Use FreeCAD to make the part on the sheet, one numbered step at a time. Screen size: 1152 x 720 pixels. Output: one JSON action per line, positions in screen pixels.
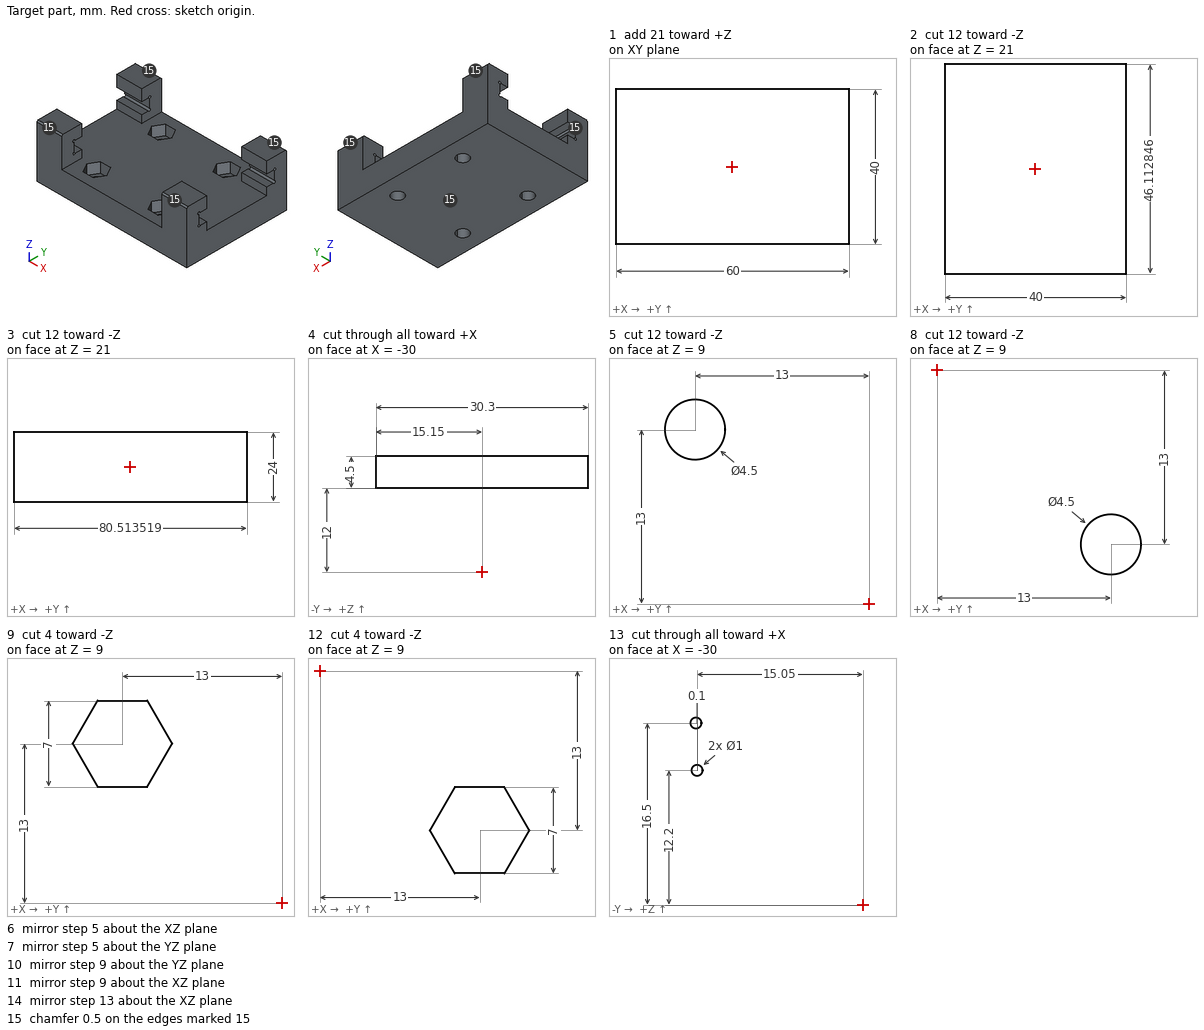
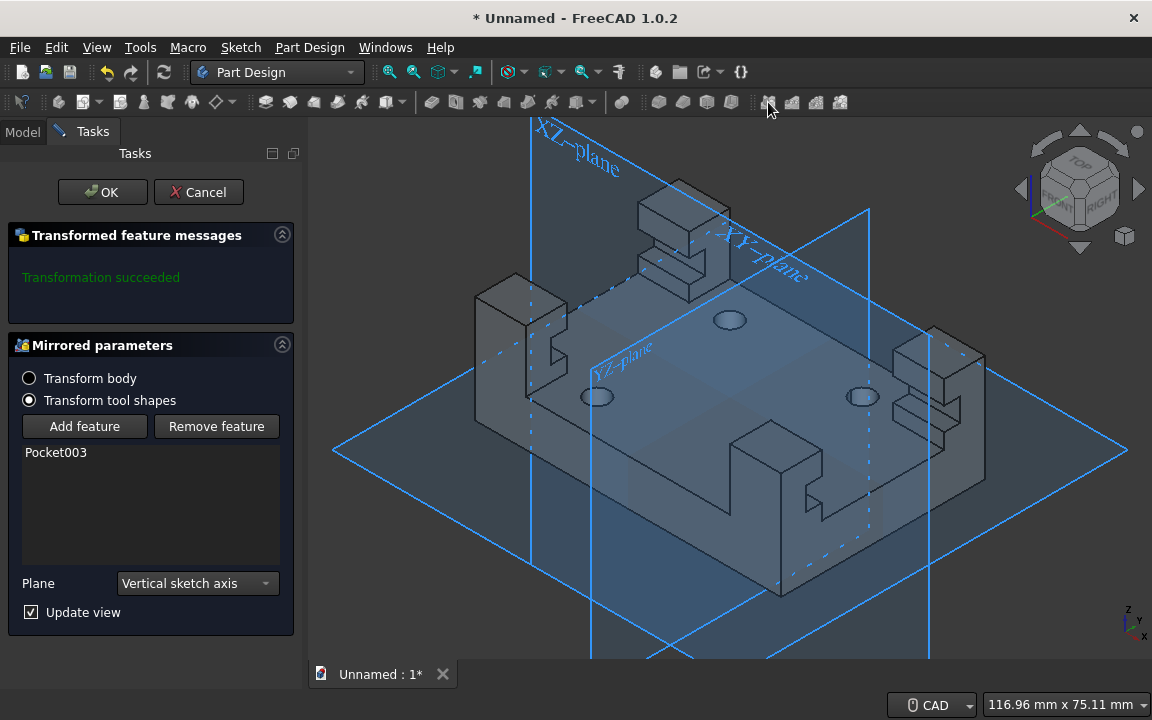
{"action": "left_click", "coordinate": [198, 584]}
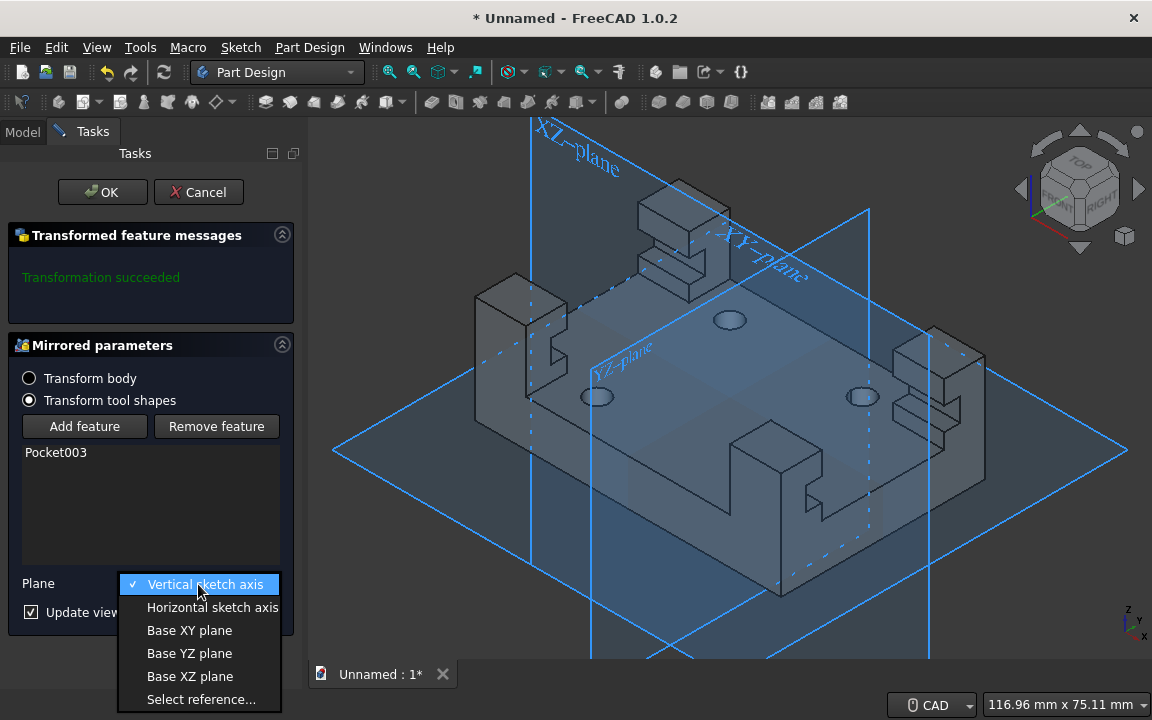
{"action": "left_click", "coordinate": [198, 654]}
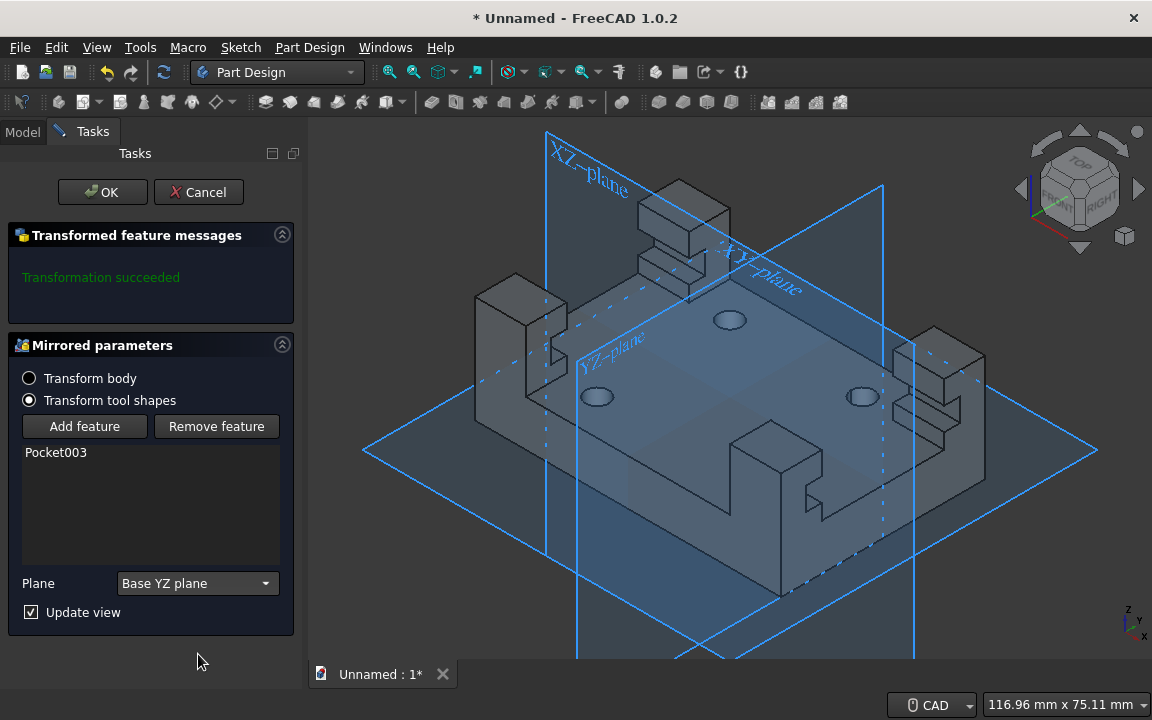
{"action": "left_click", "coordinate": [103, 192]}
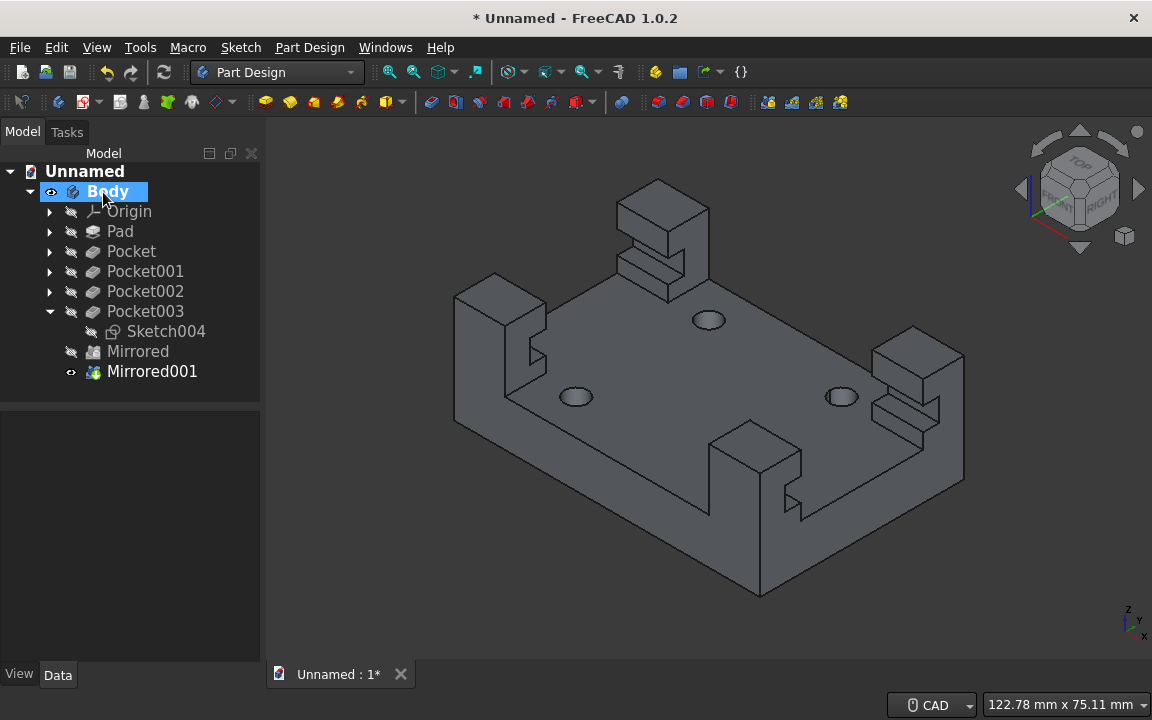
{"action": "left_click", "coordinate": [709, 396]}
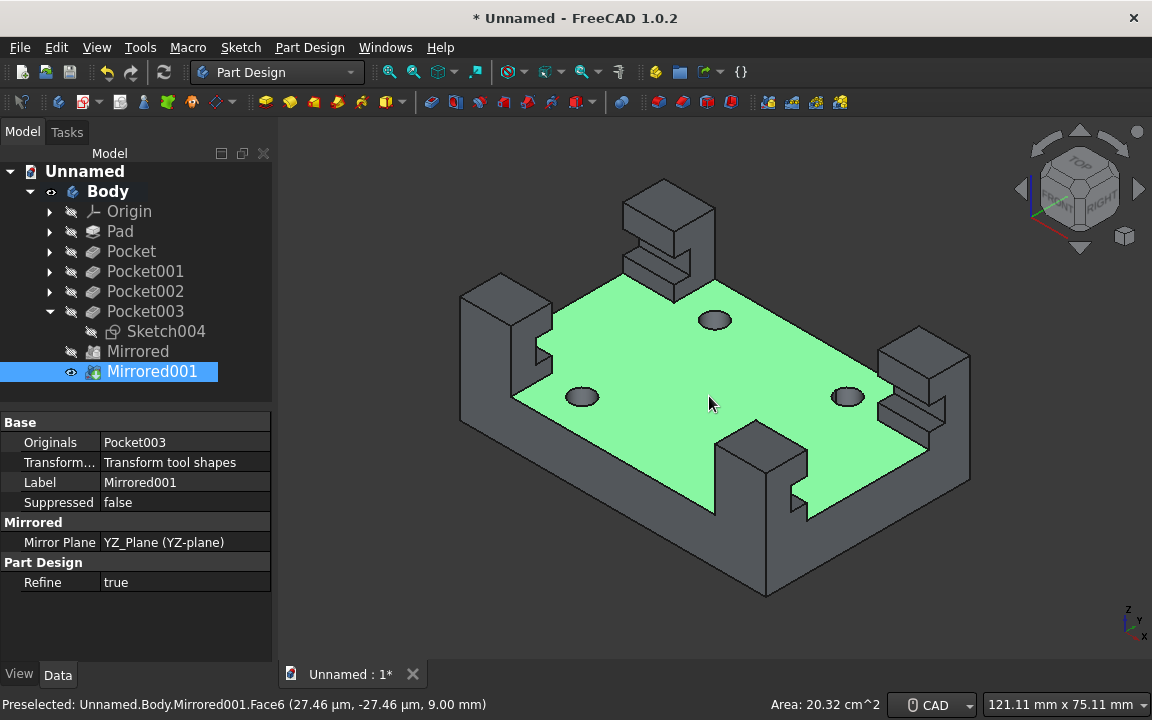
{"action": "left_click", "coordinate": [84, 102]}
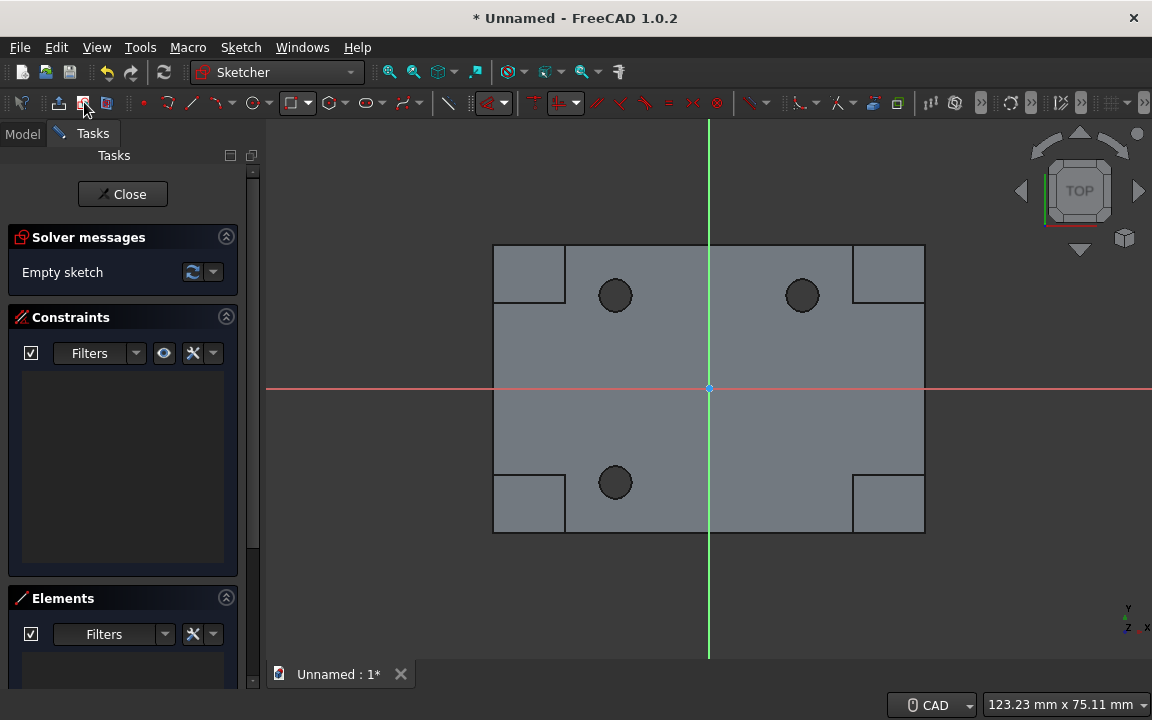
{"action": "left_click", "coordinate": [108, 104]}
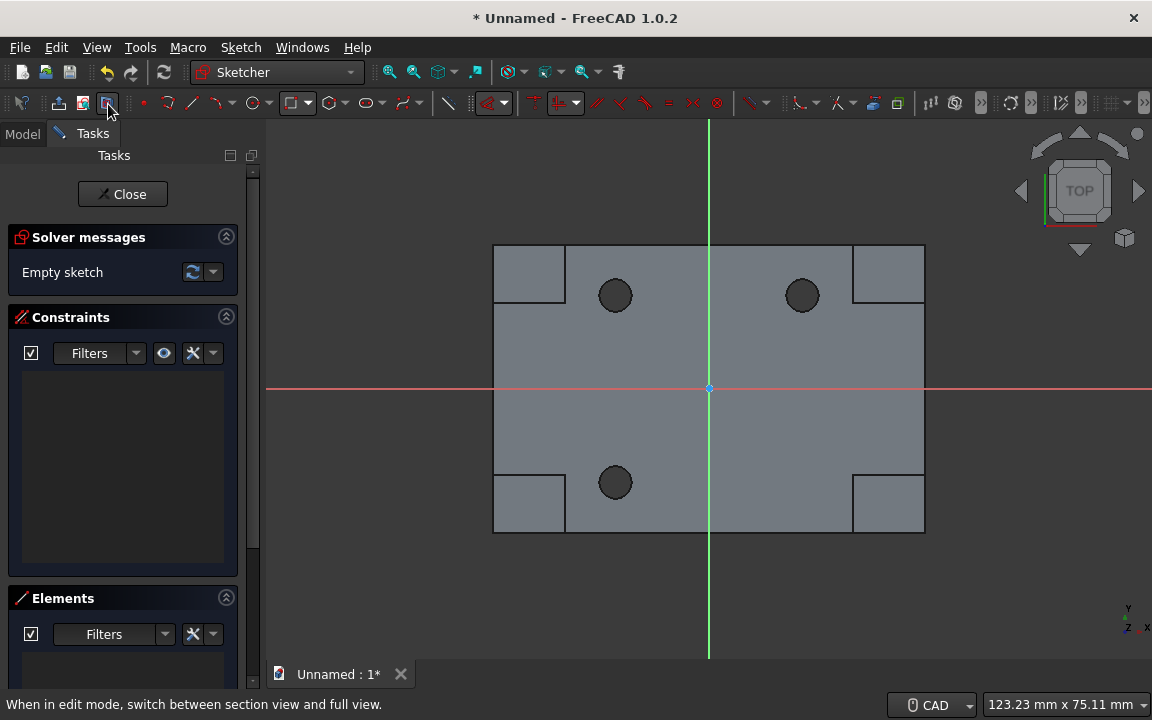
{"action": "scroll", "coordinate": [819, 492], "scroll_direction": "up", "scroll_amount": 12}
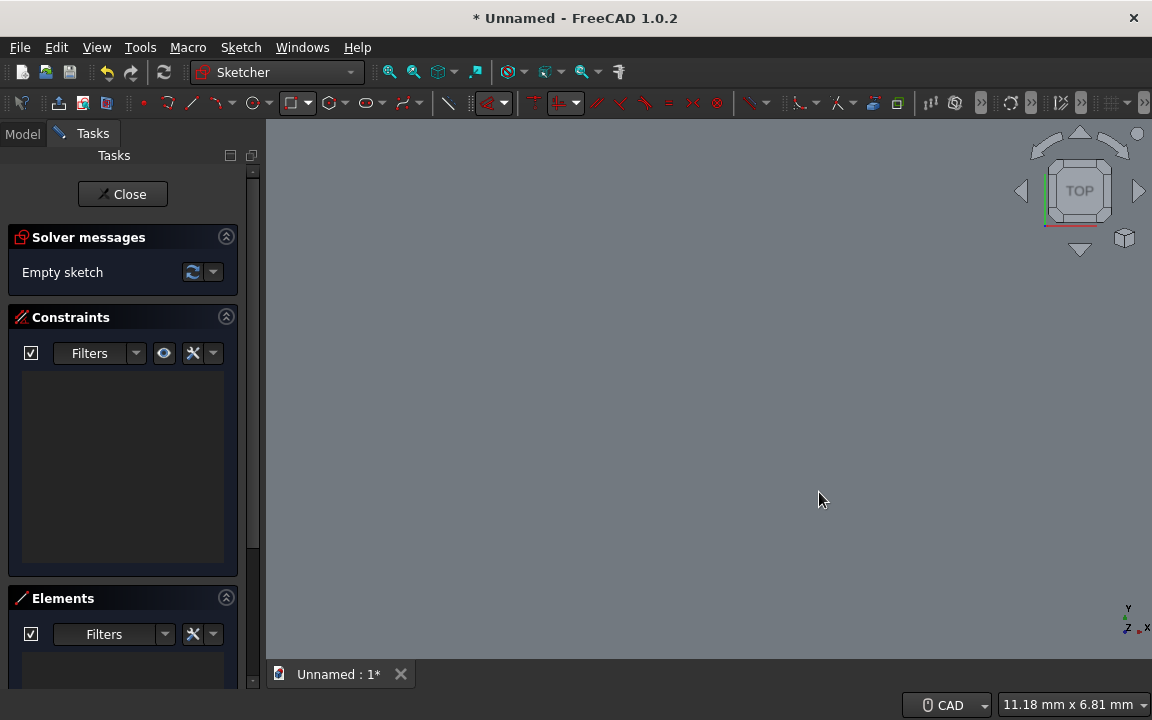
{"action": "left_click", "coordinate": [254, 104]}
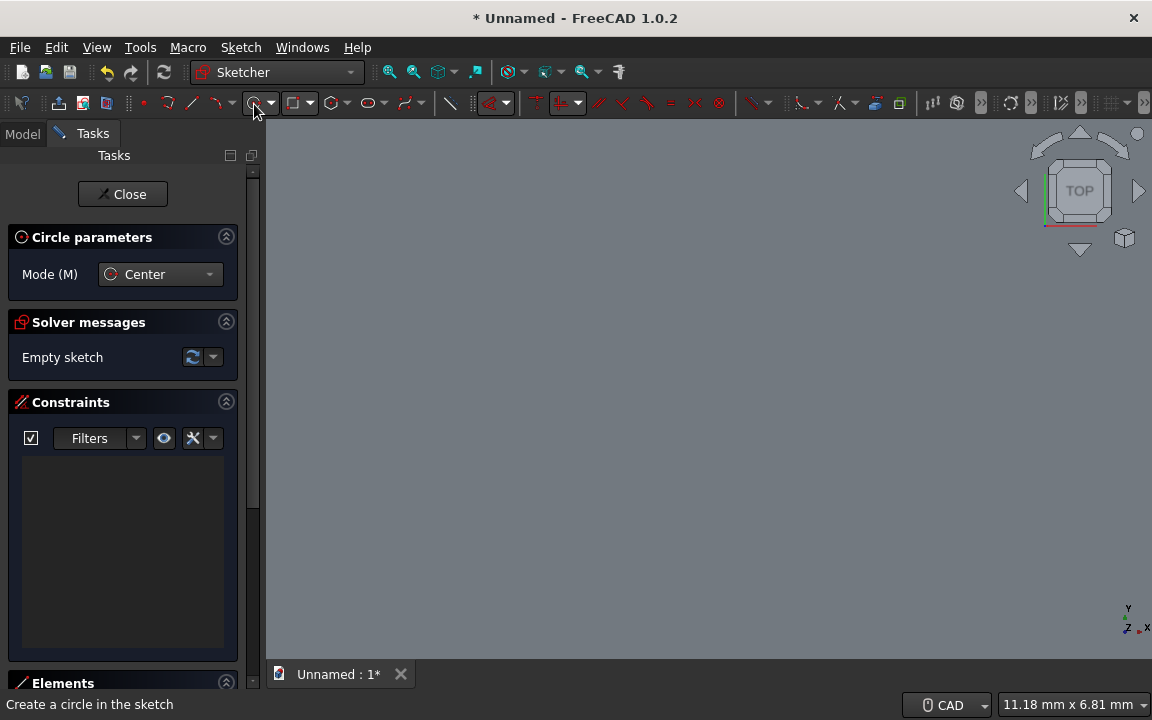
{"action": "left_click", "coordinate": [630, 380]}
{"action": "left_click", "coordinate": [757, 254]}
{"action": "key", "text": "Escape"}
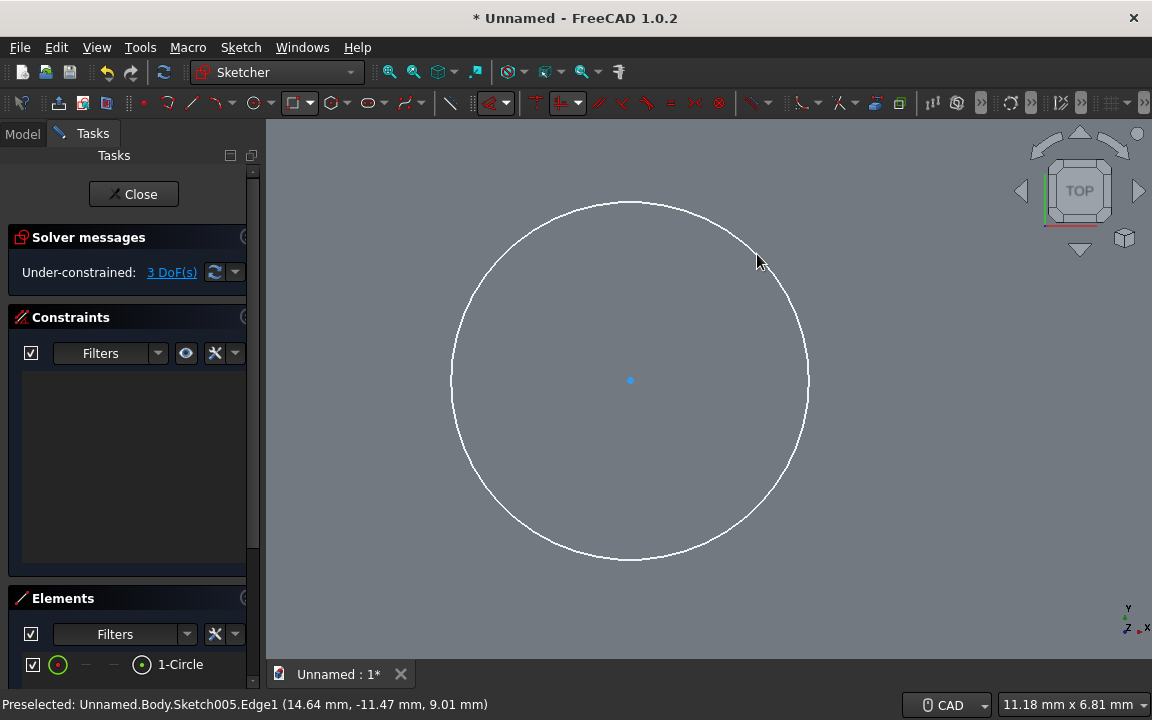
{"action": "left_click", "coordinate": [756, 254]}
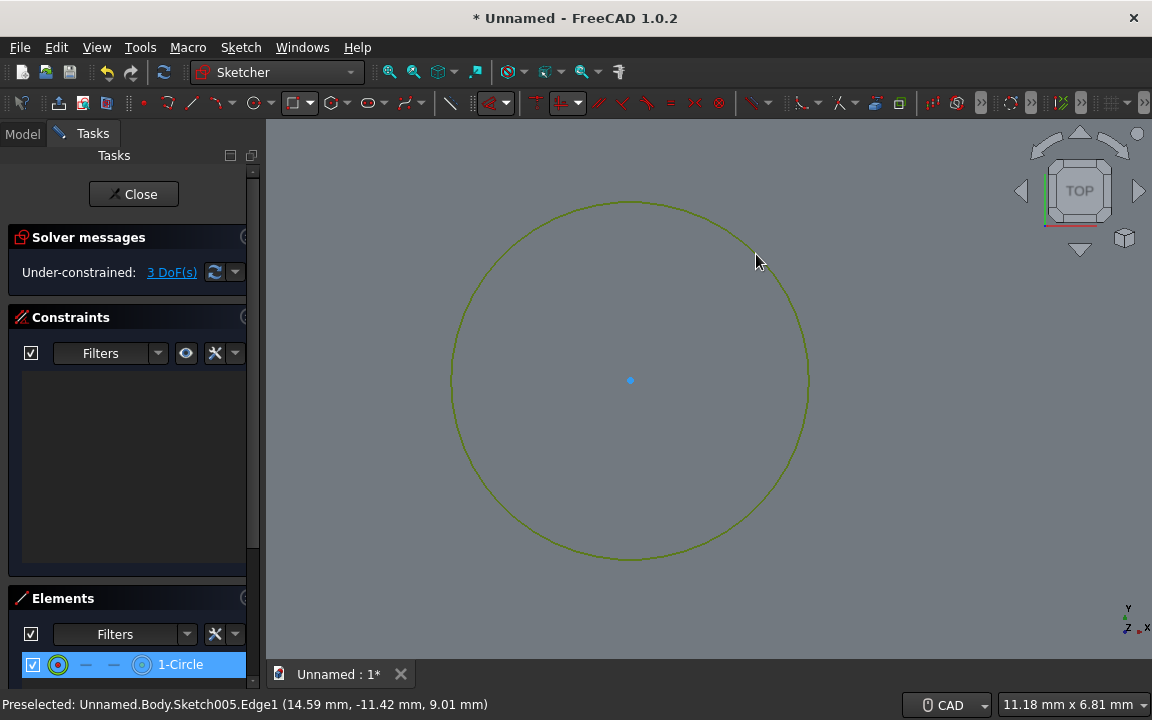
{"action": "left_click", "coordinate": [508, 104]}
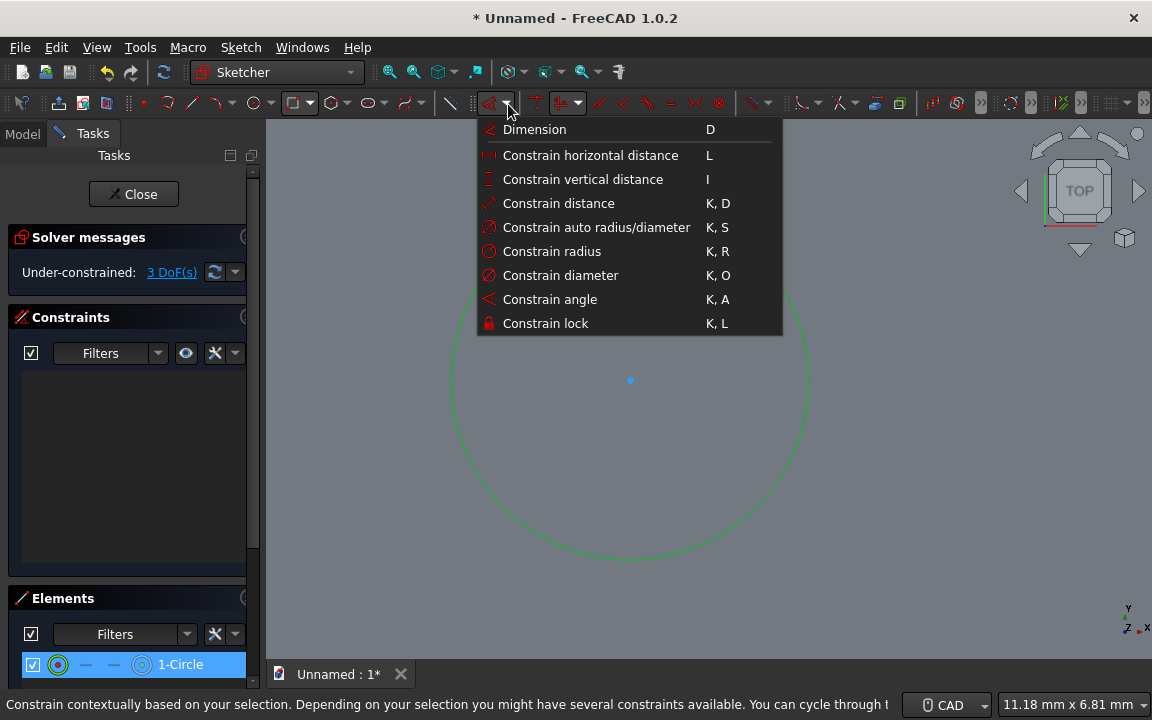
{"action": "left_click", "coordinate": [630, 275]}